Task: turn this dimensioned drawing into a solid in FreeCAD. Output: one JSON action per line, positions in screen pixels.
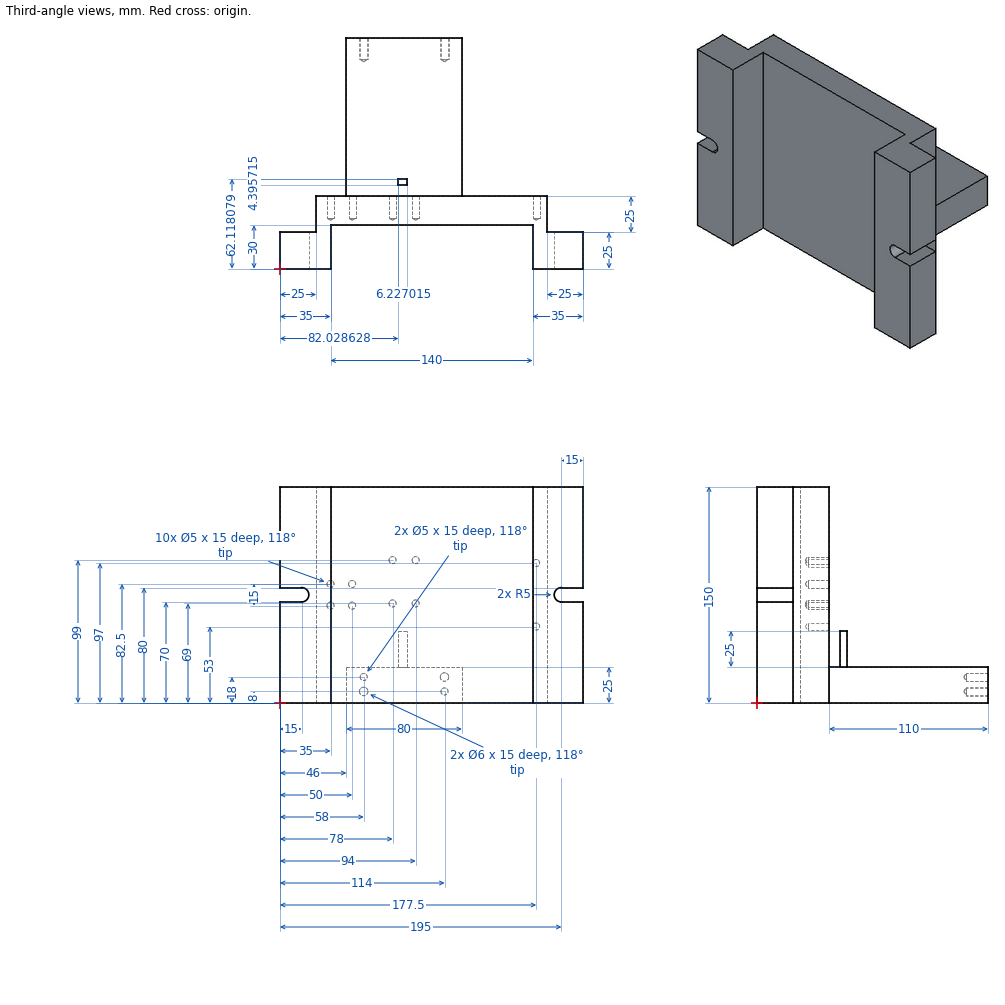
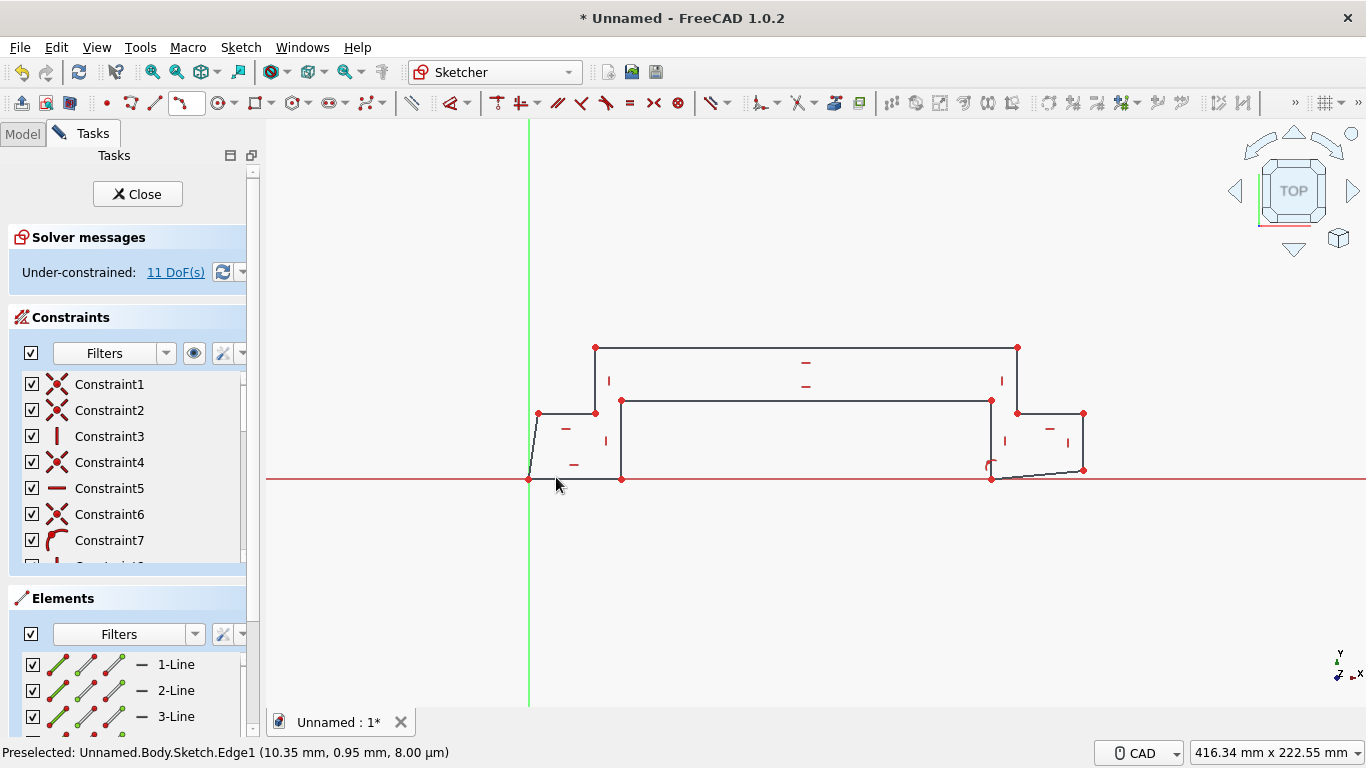
{"action": "left_click", "coordinate": [1019, 477]}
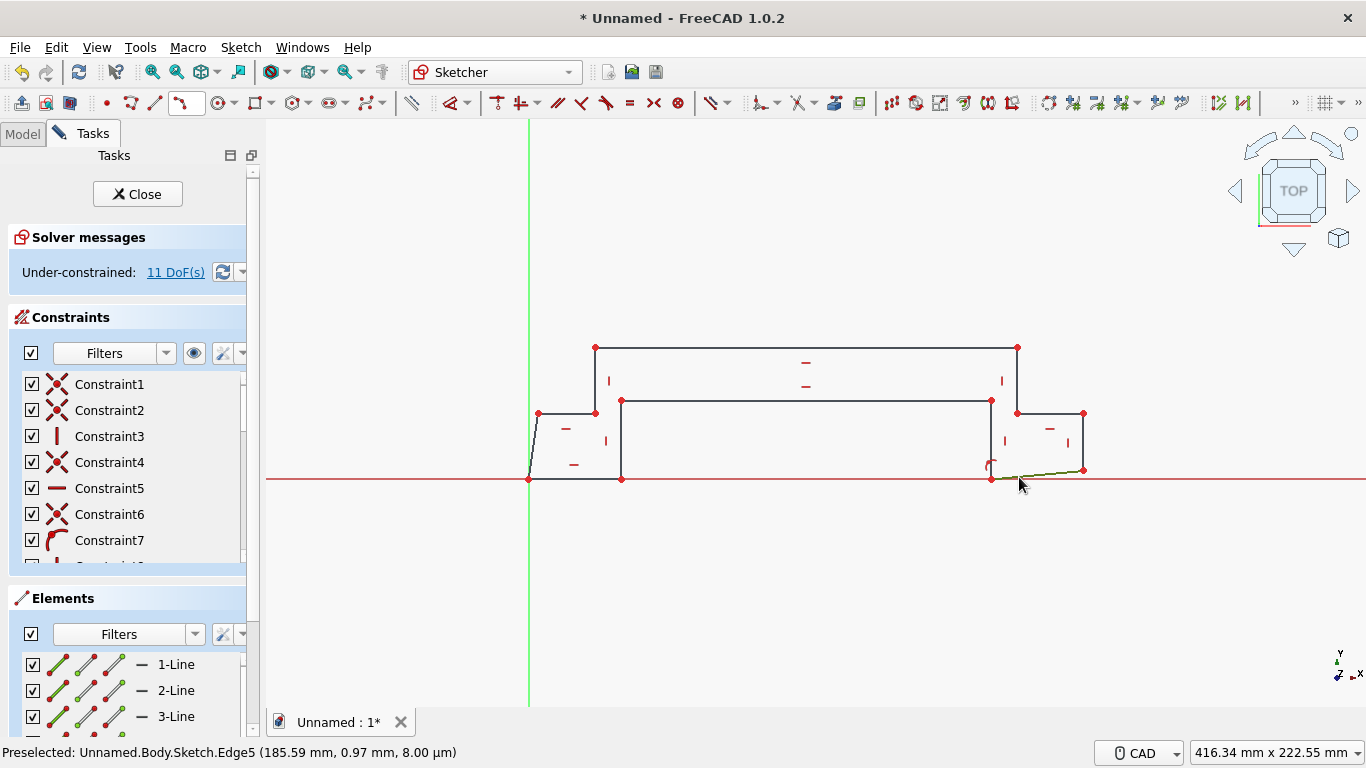
{"action": "key", "text": "h"}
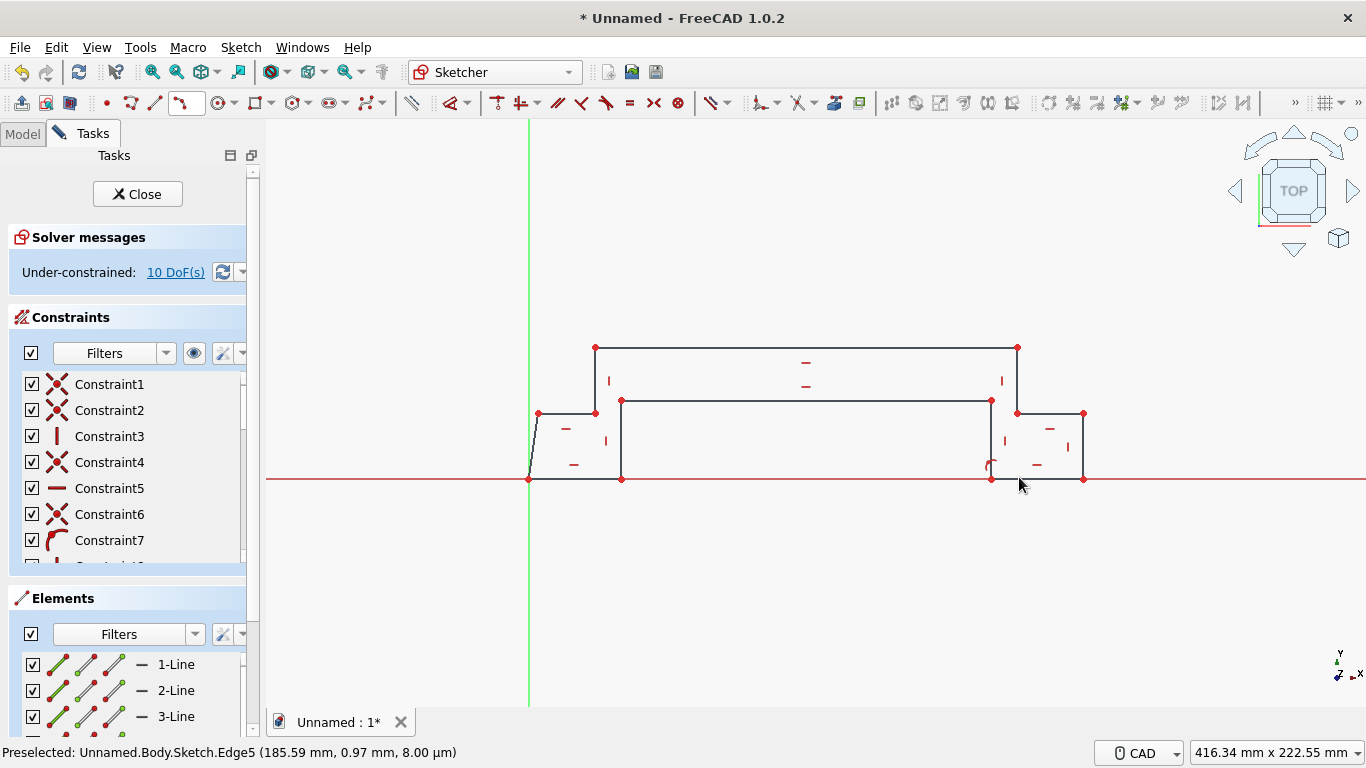
{"action": "left_click", "coordinate": [531, 460]}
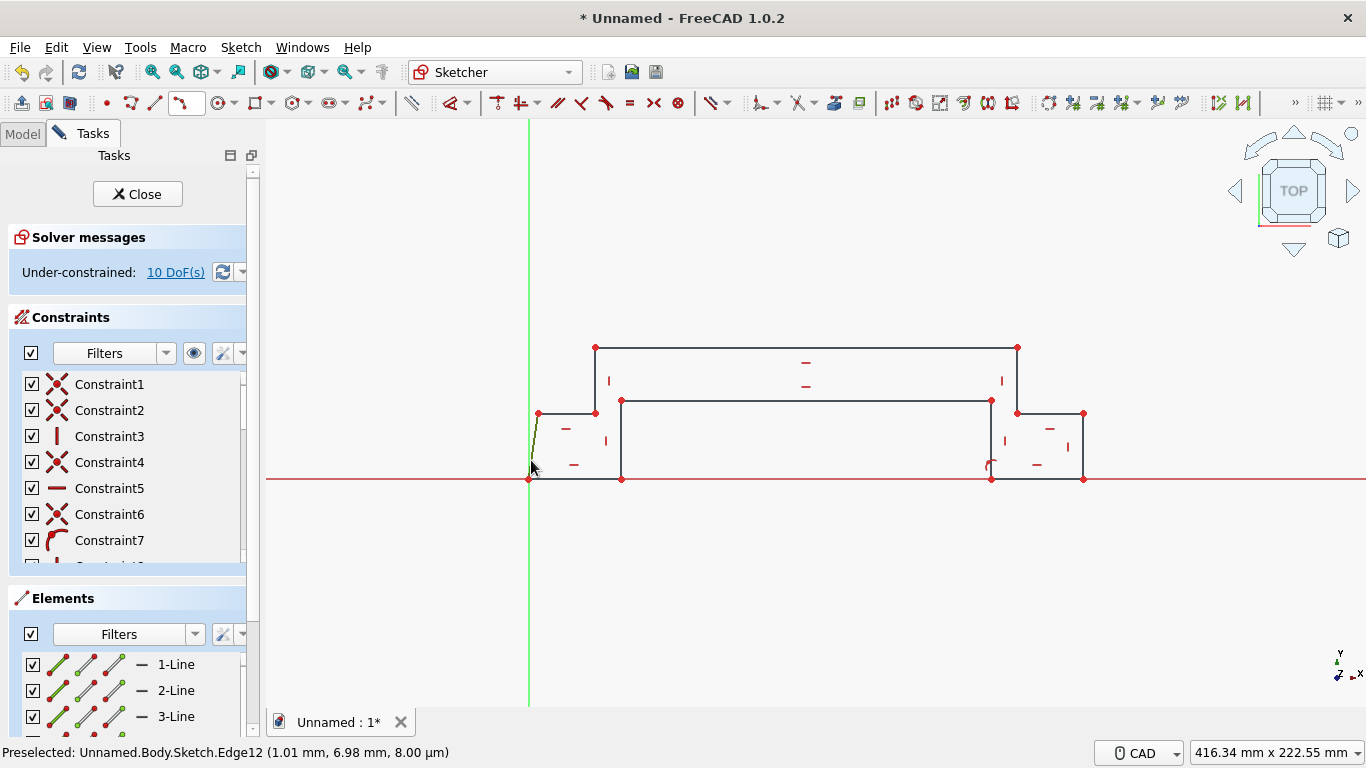
{"action": "key", "text": "v"}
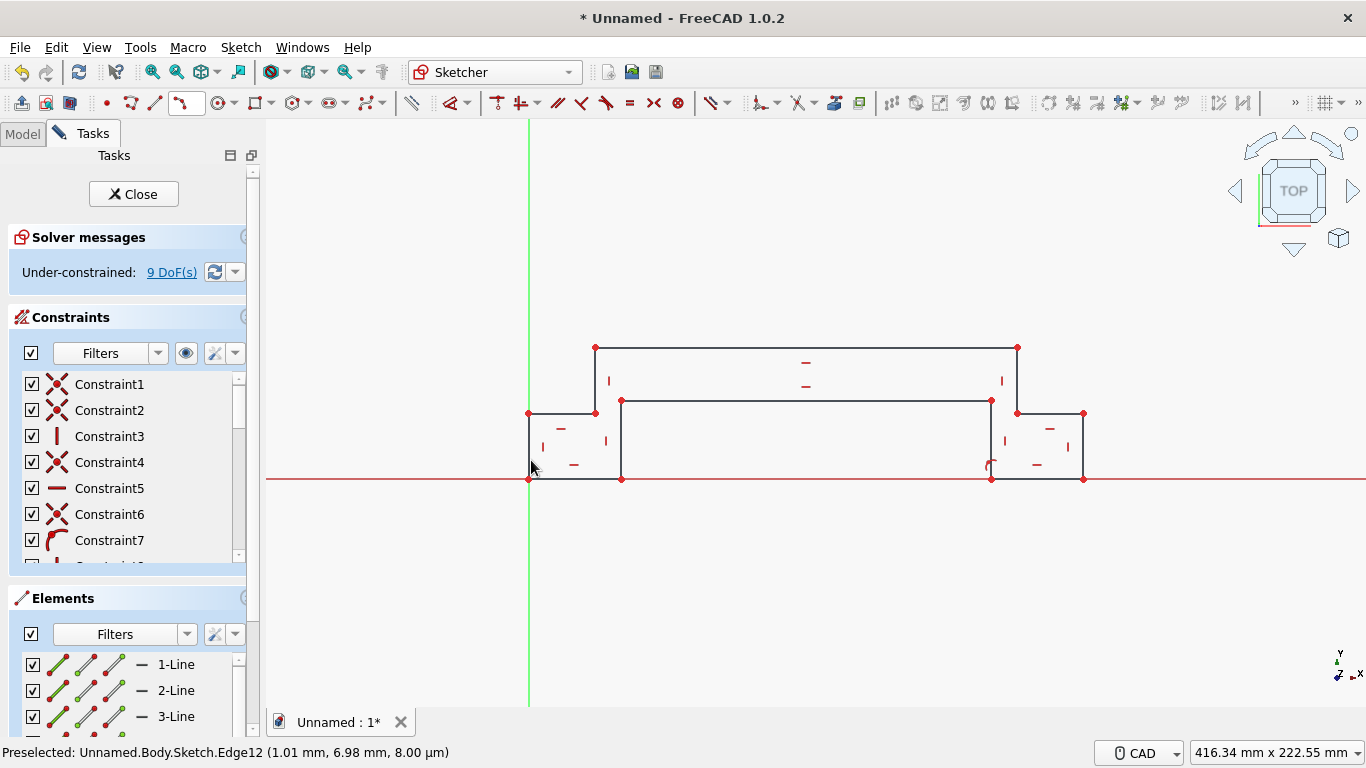
{"action": "left_click", "coordinate": [450, 104]}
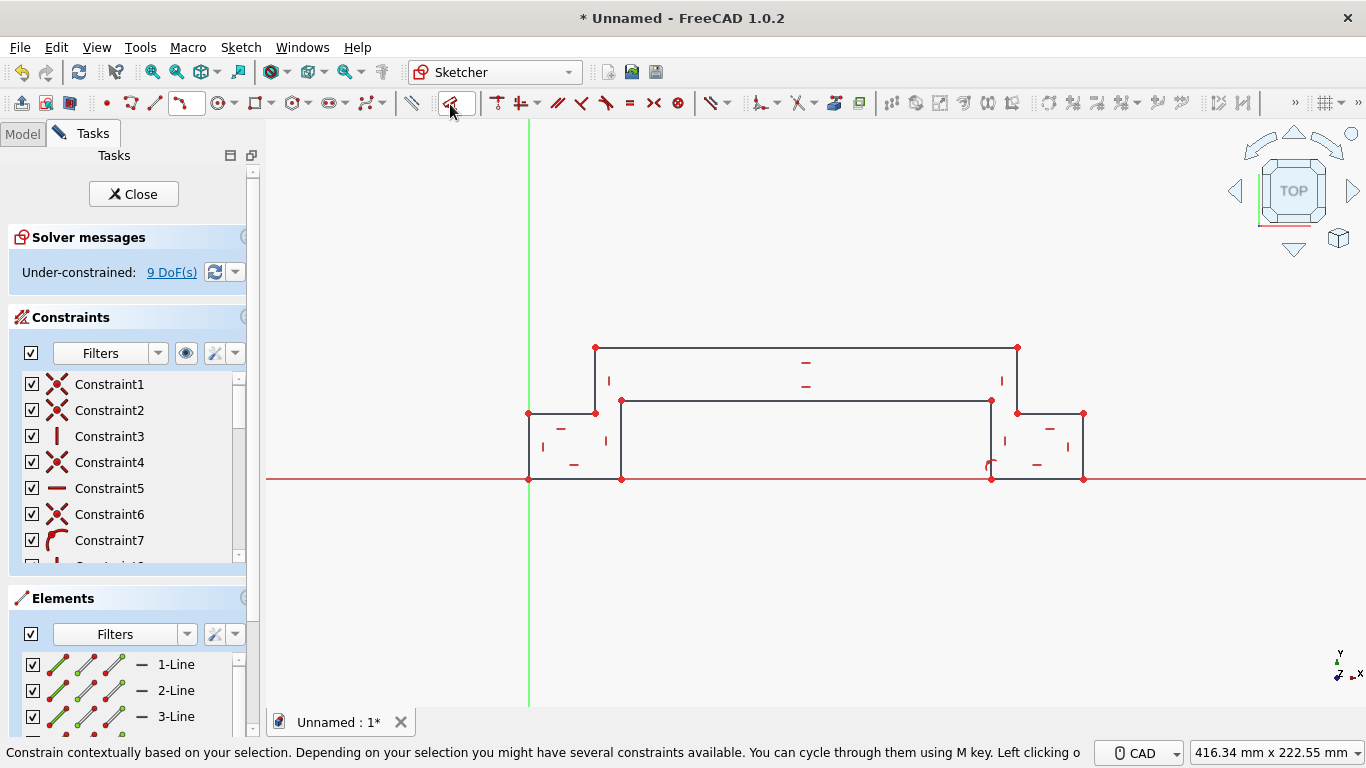
{"action": "left_click", "coordinate": [556, 479]}
{"action": "left_click", "coordinate": [575, 513]}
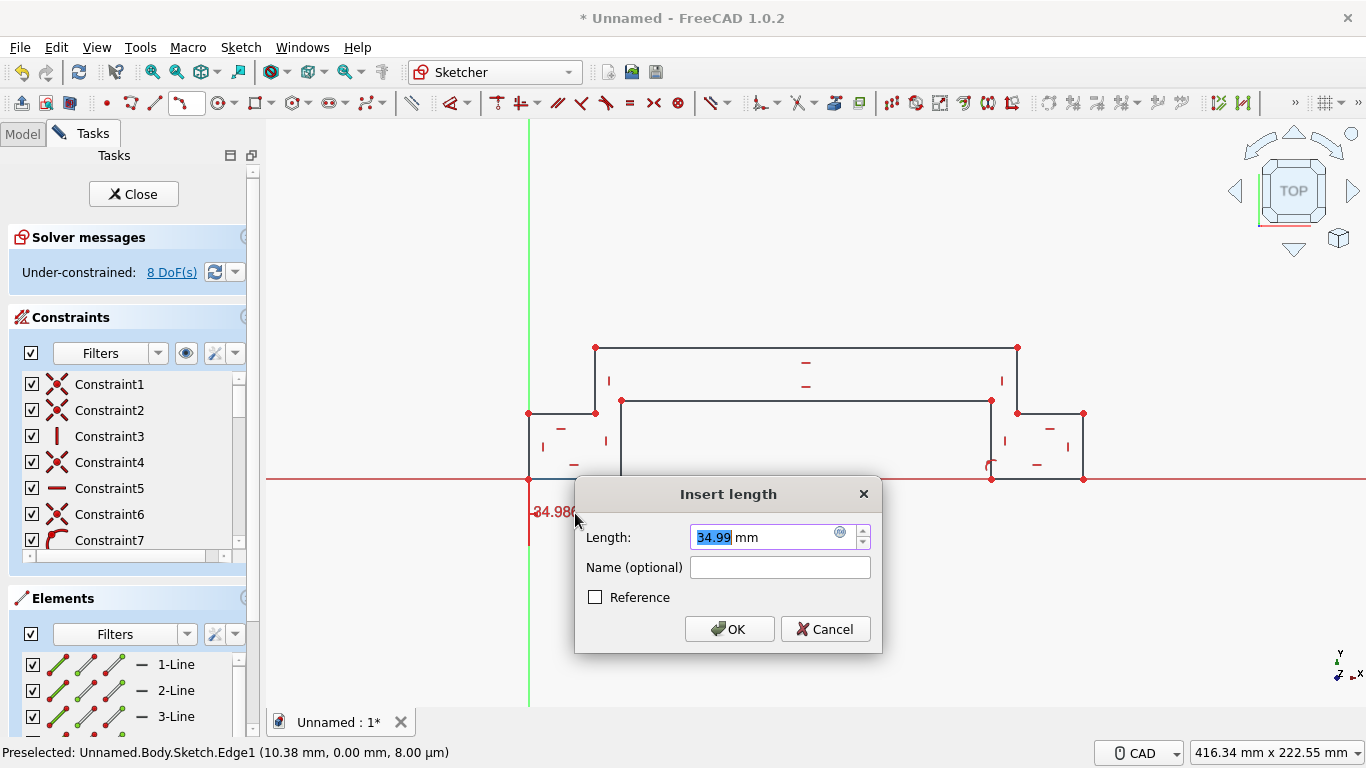
{"action": "type", "text": "35"}
{"action": "key", "text": "Return"}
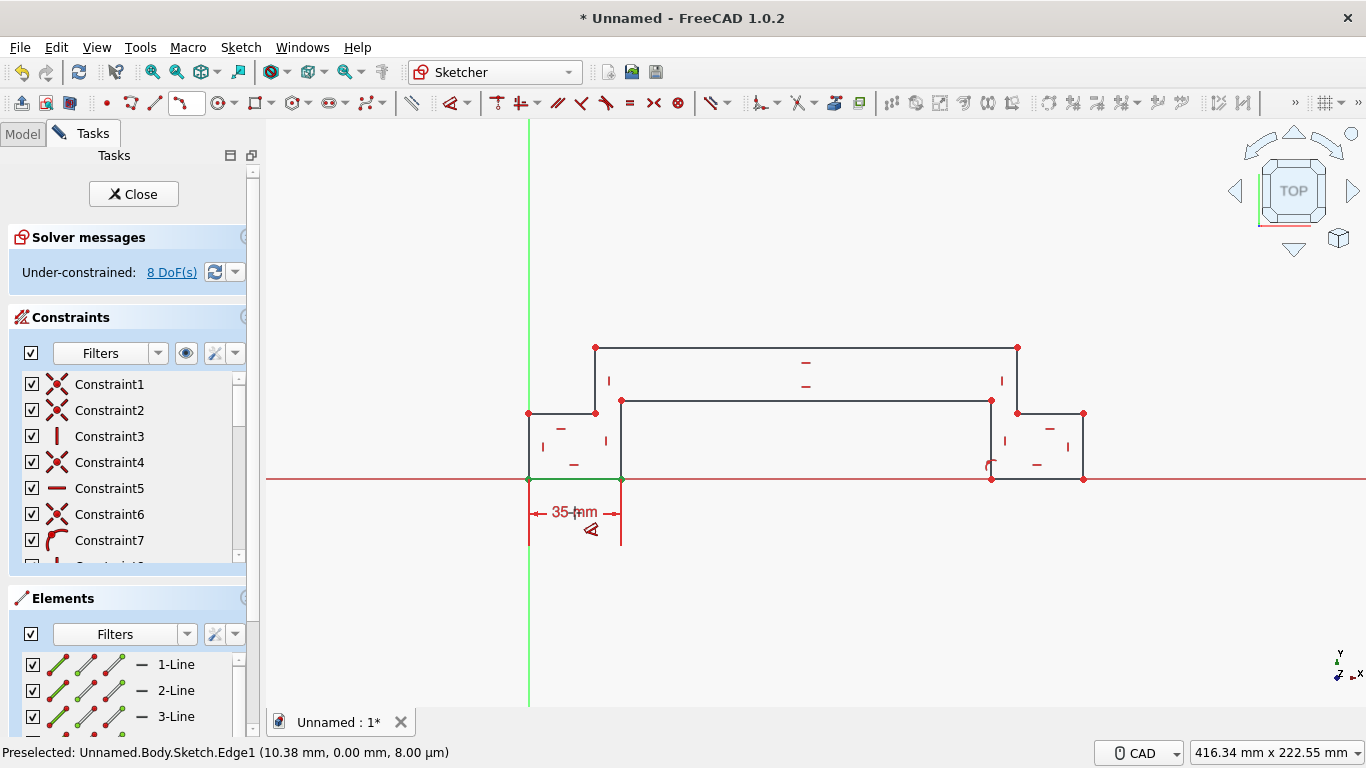
{"action": "left_click", "coordinate": [621, 456]}
{"action": "left_click", "coordinate": [587, 440]}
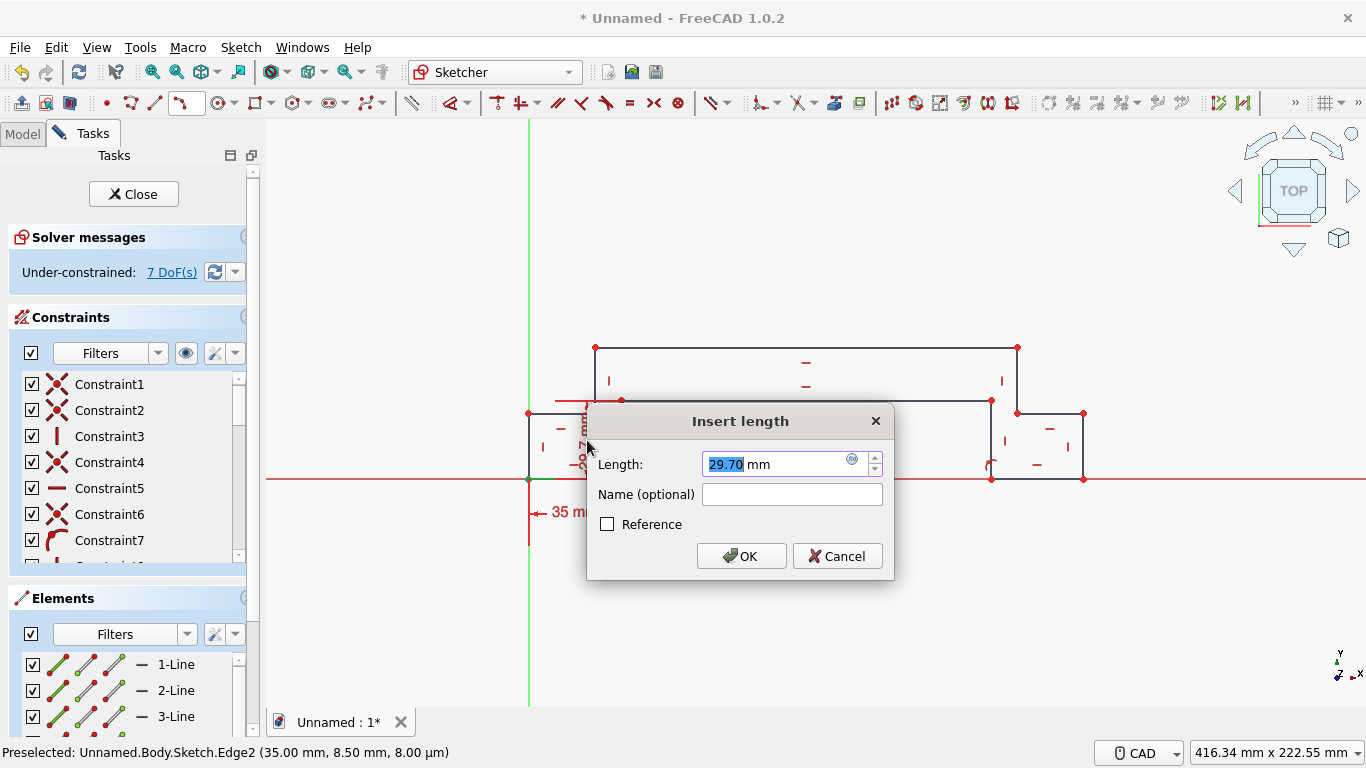
{"action": "type", "text": "30"}
{"action": "key", "text": "Return"}